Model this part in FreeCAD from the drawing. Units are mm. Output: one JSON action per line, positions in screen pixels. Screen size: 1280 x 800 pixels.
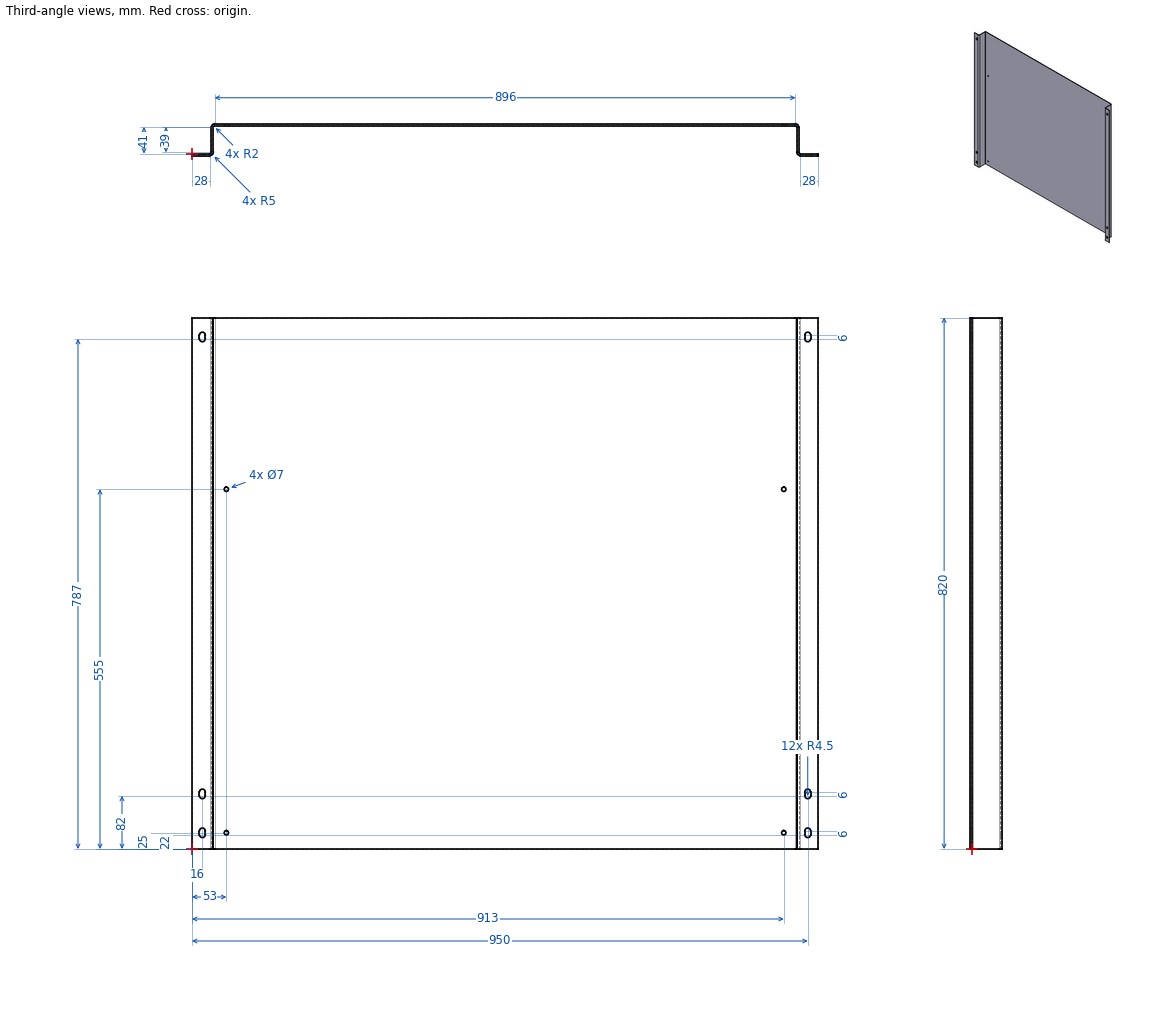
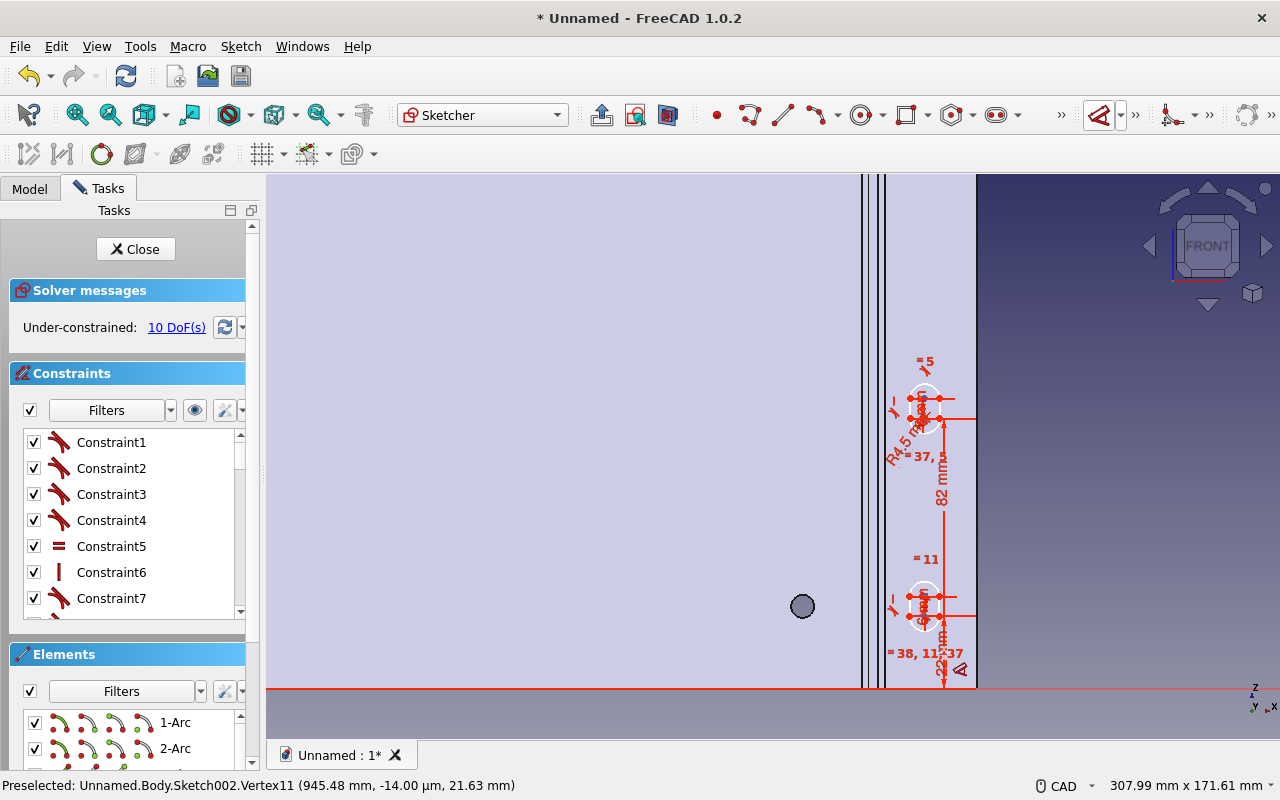
{"action": "scroll", "coordinate": [914, 626], "scroll_direction": "down", "scroll_amount": 10}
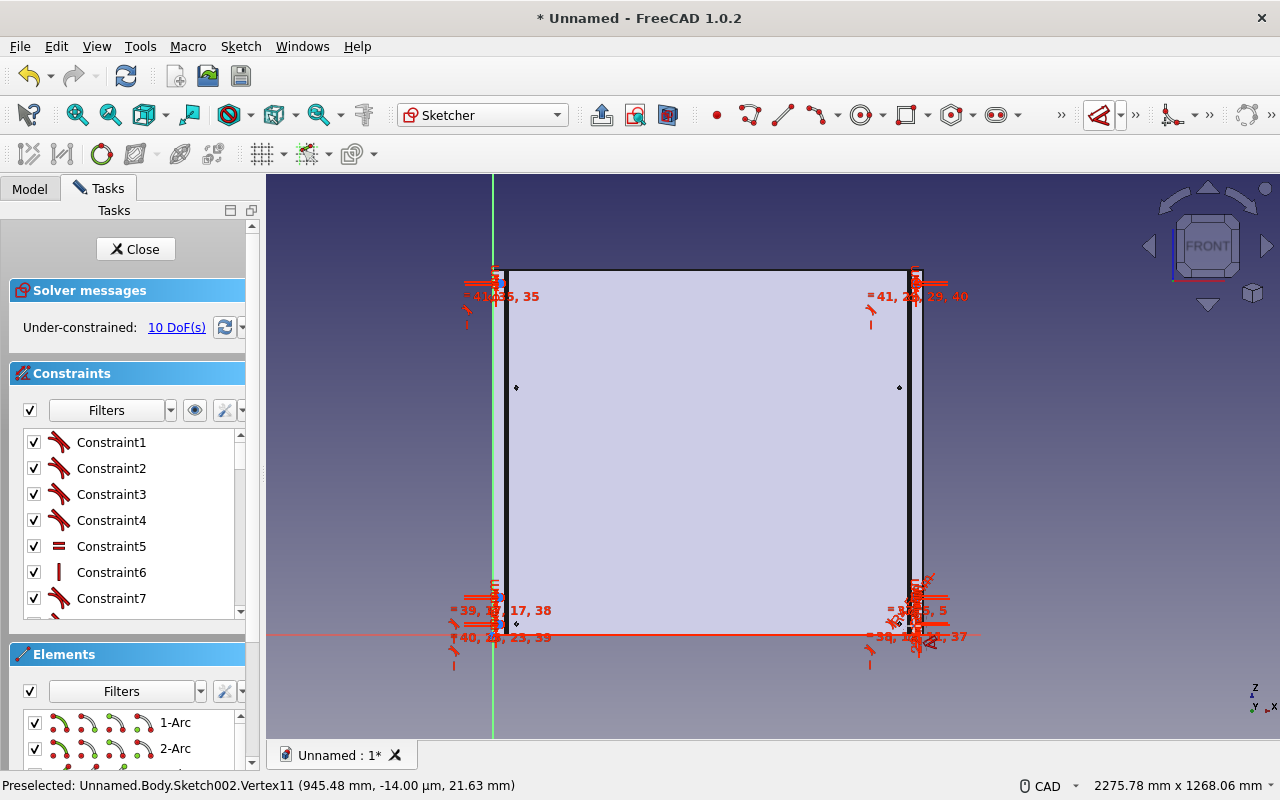
{"action": "scroll", "coordinate": [498, 599], "scroll_direction": "up", "scroll_amount": 10}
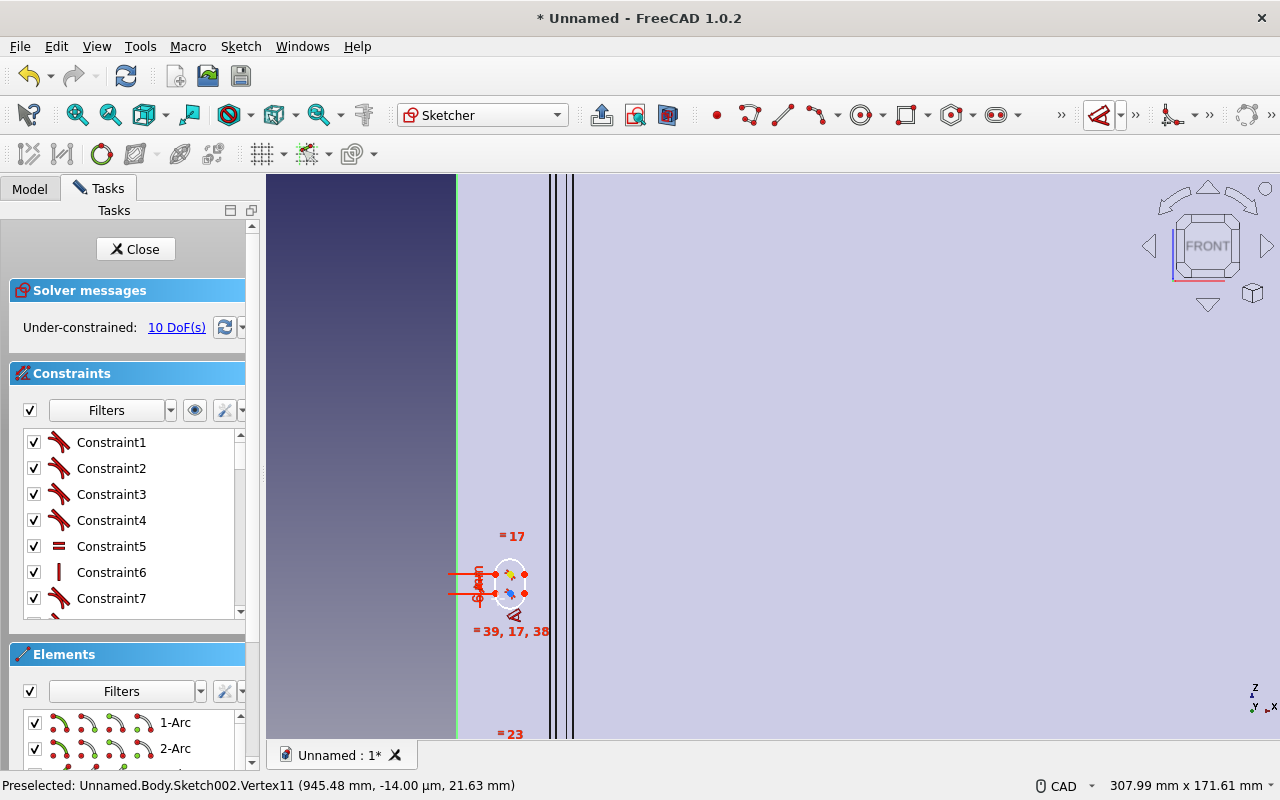
{"action": "left_click", "coordinate": [495, 594]}
{"action": "left_click", "coordinate": [423, 652]}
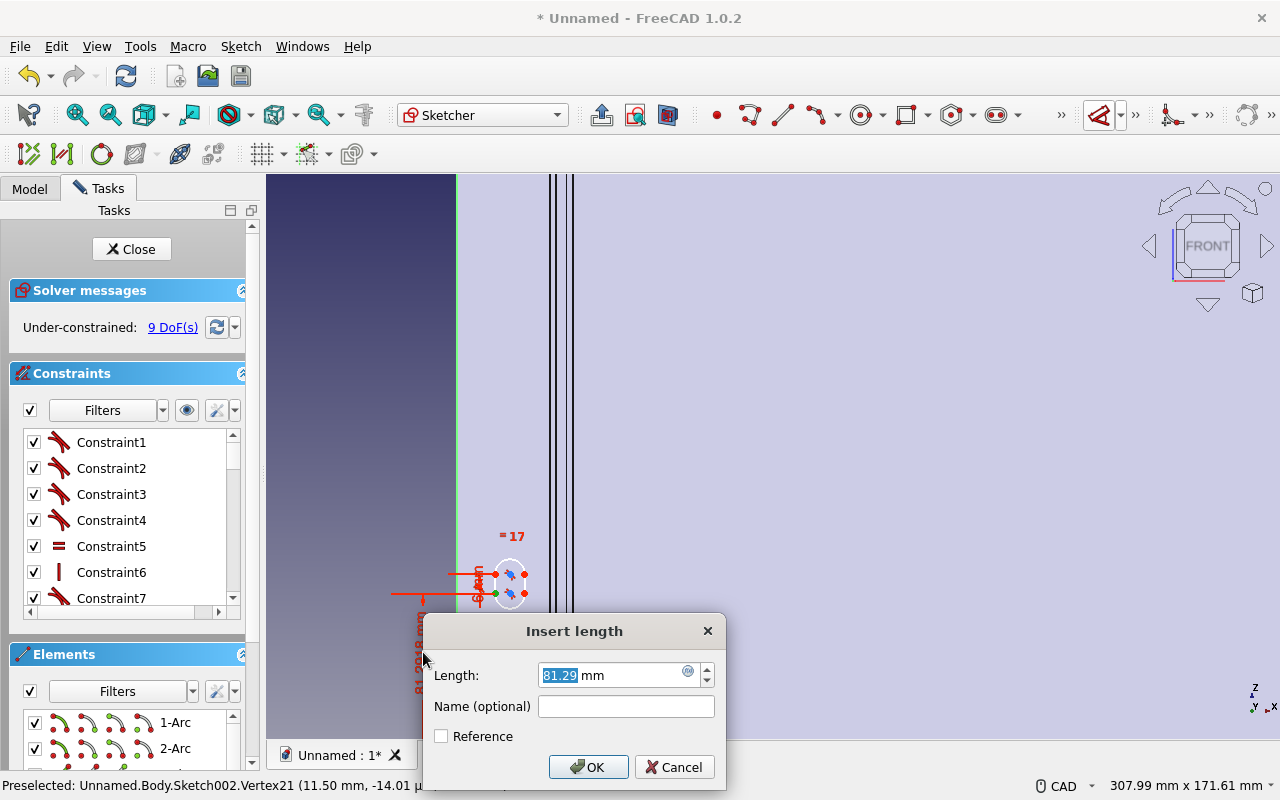
{"action": "type", "text": "82"}
{"action": "key", "text": "Return"}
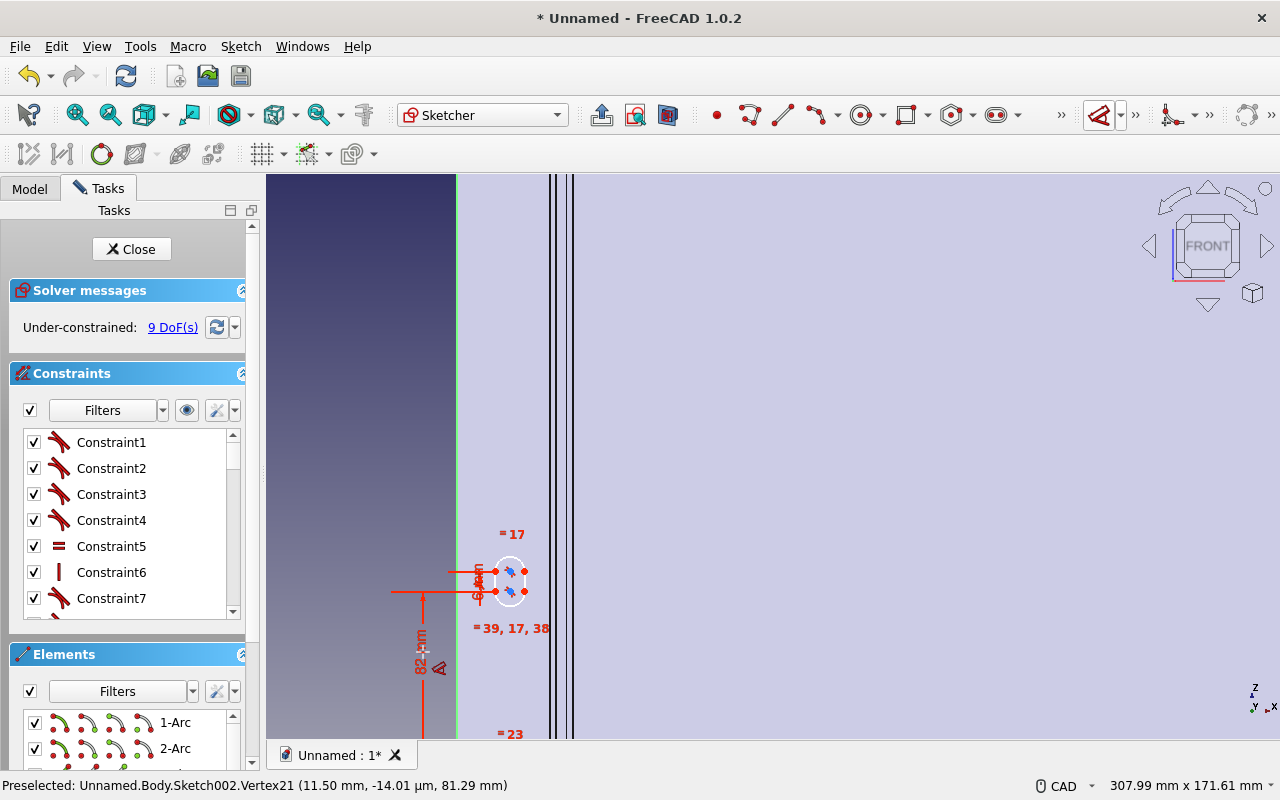
{"action": "scroll", "coordinate": [497, 599], "scroll_direction": "down", "scroll_amount": 10}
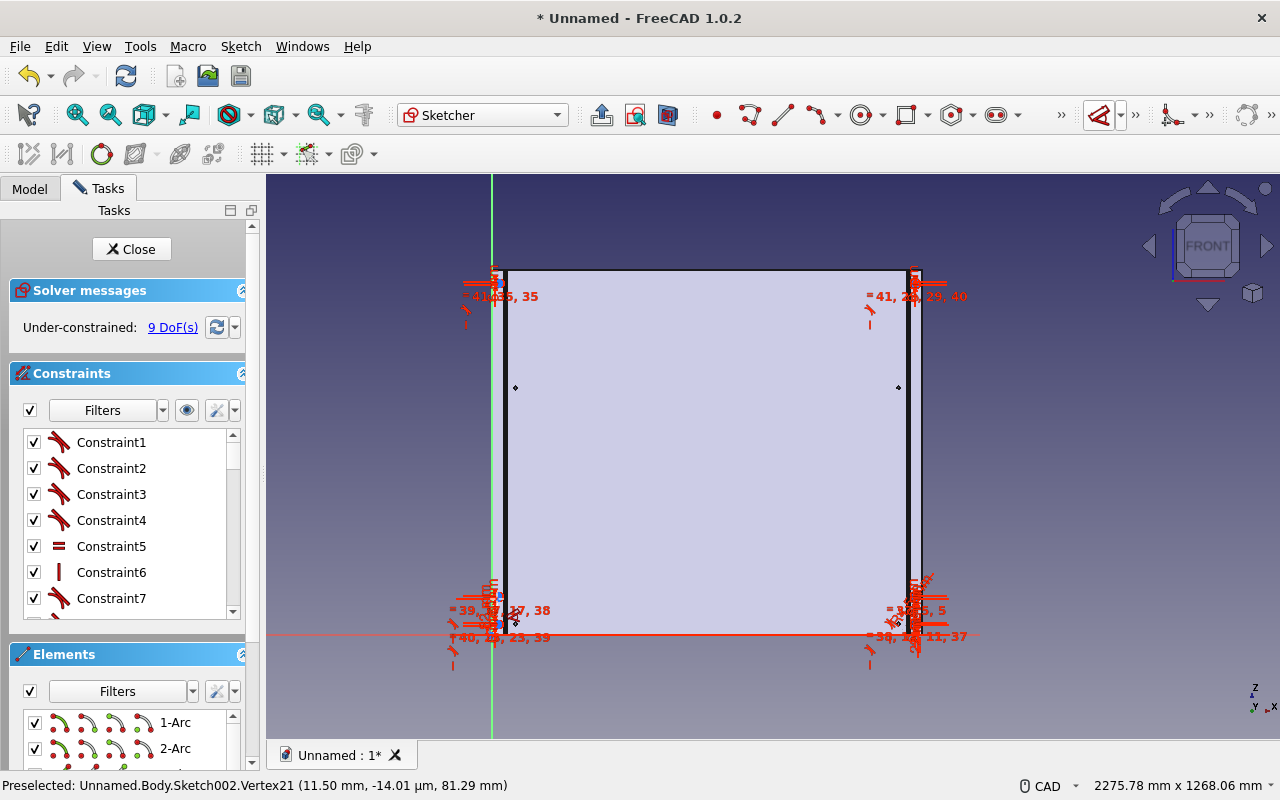
{"action": "scroll", "coordinate": [497, 626], "scroll_direction": "up", "scroll_amount": 10}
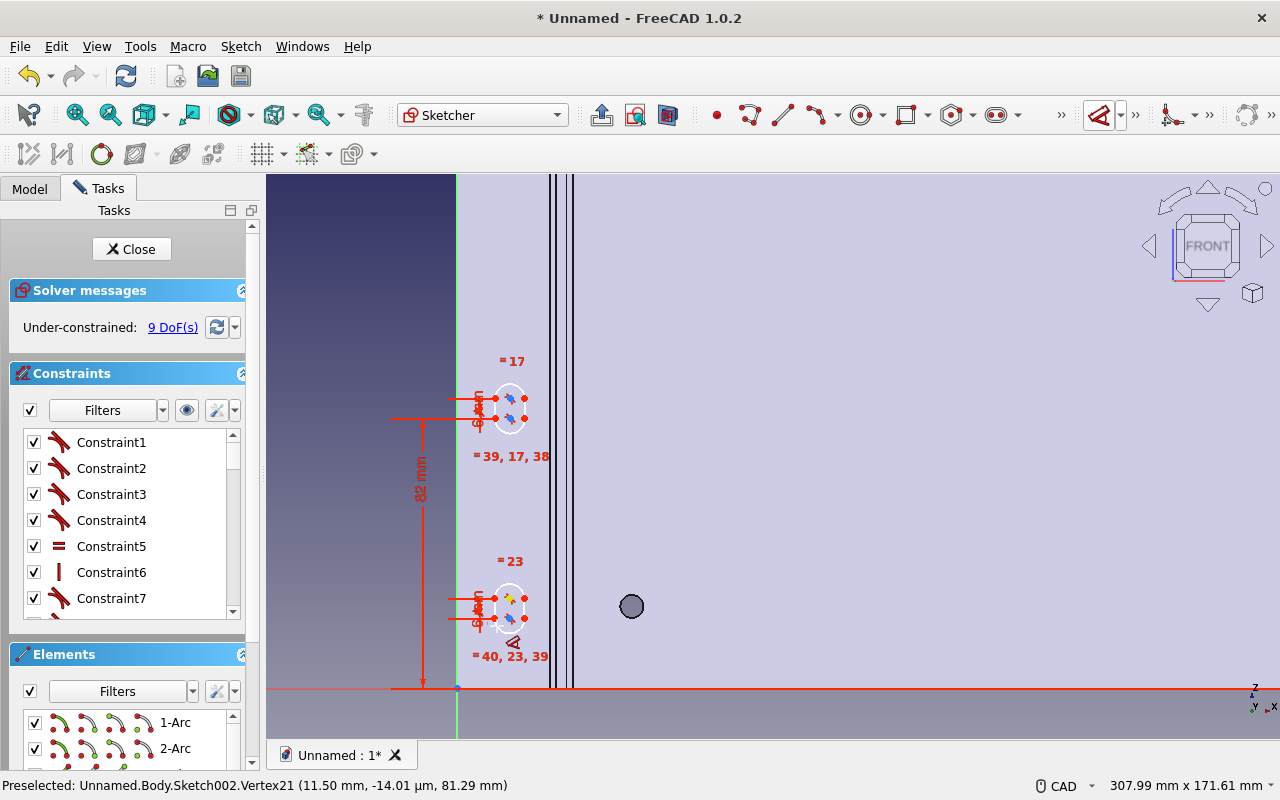
{"action": "left_click", "coordinate": [495, 619]}
{"action": "left_click", "coordinate": [423, 654]}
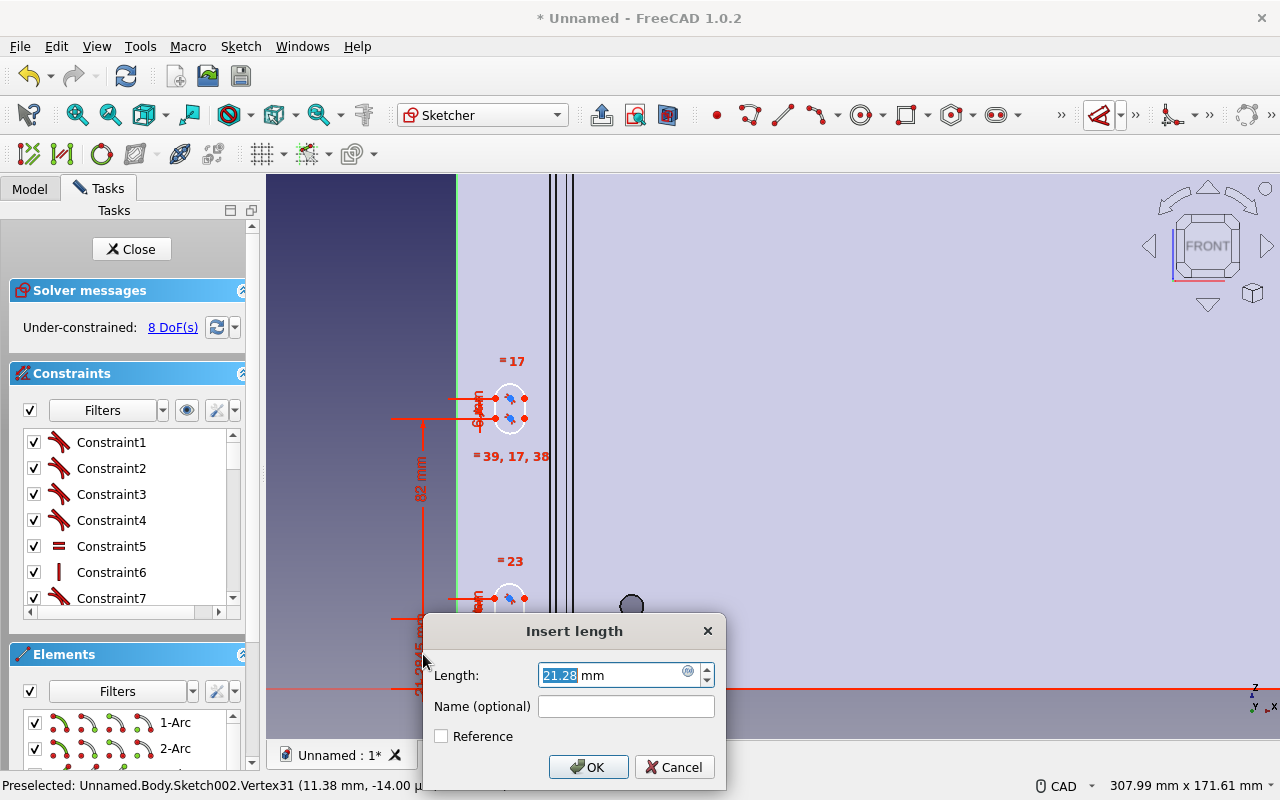
{"action": "type", "text": "22"}
{"action": "key", "text": "Return"}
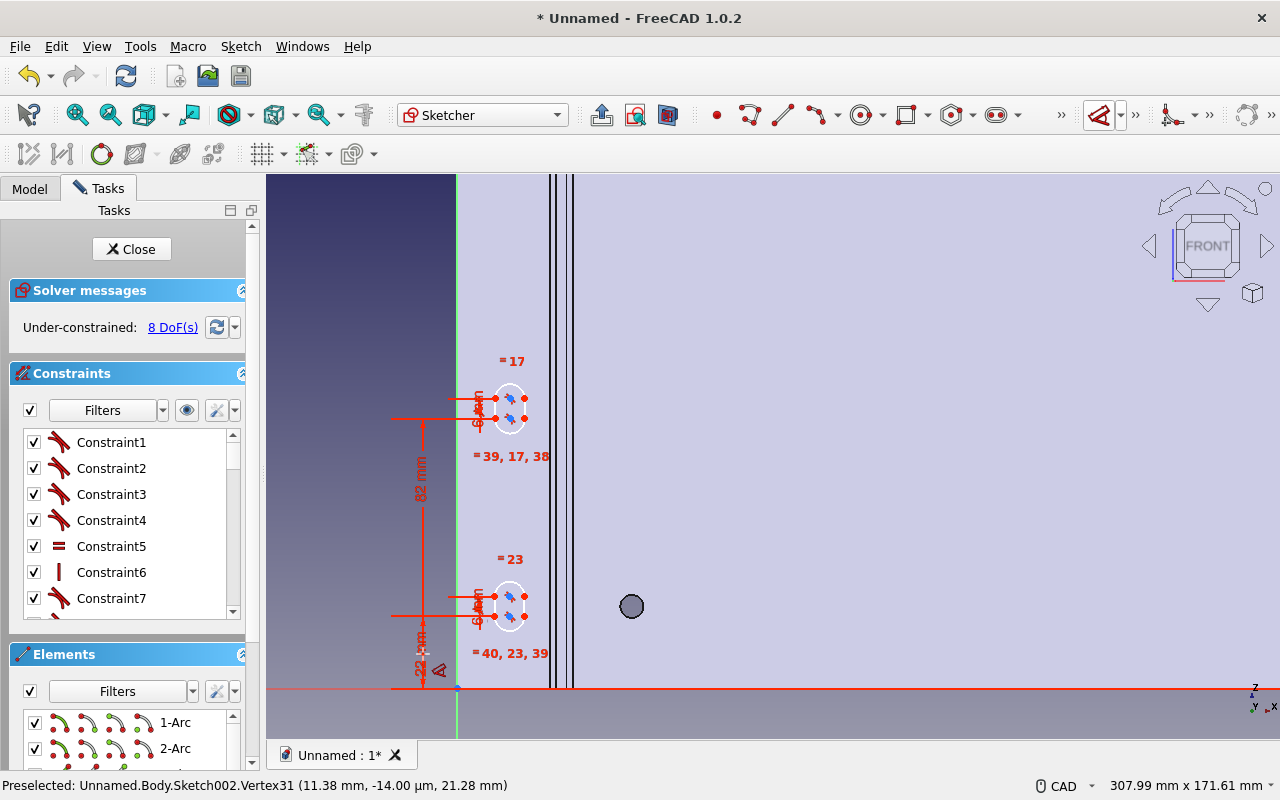
{"action": "left_click", "coordinate": [510, 419]}
{"action": "left_click", "coordinate": [484, 385]}